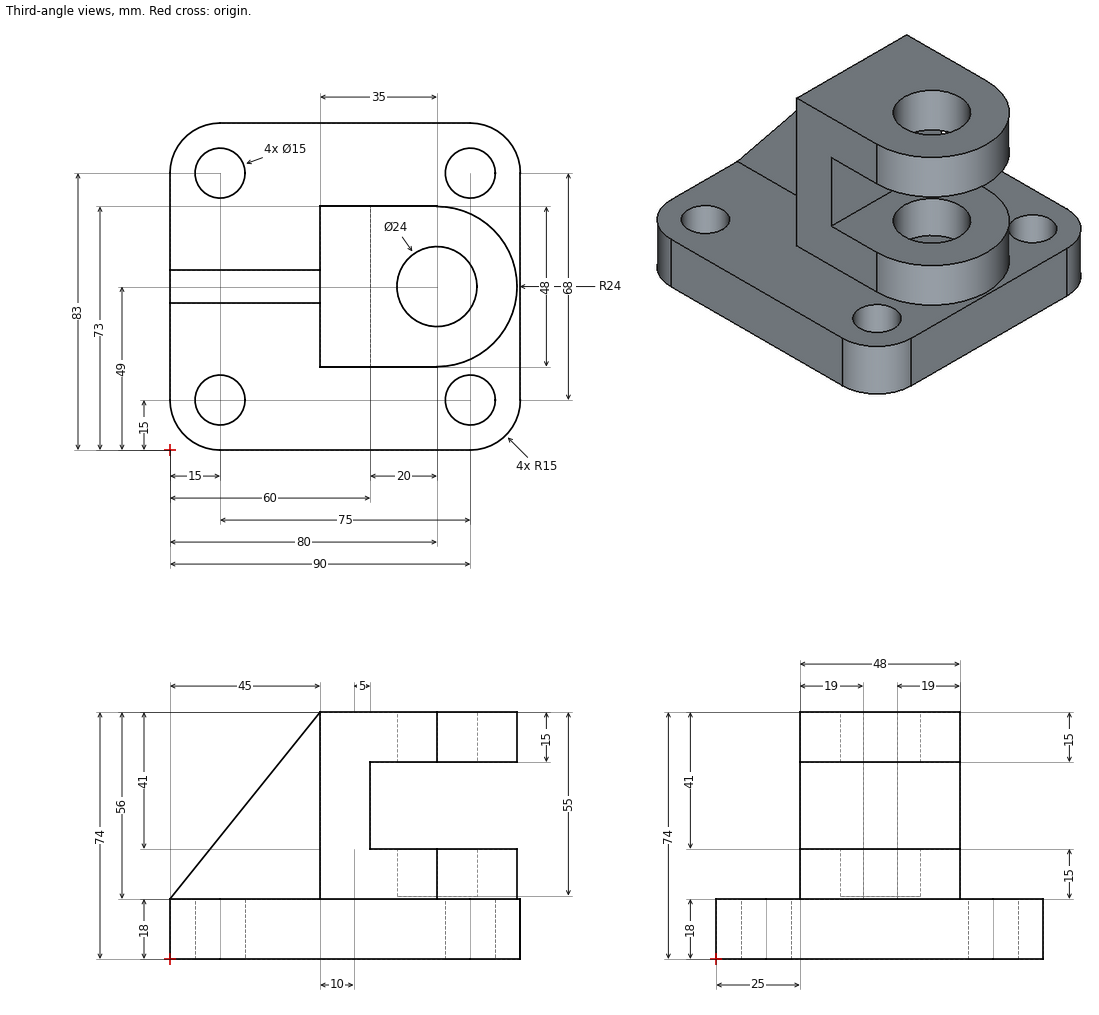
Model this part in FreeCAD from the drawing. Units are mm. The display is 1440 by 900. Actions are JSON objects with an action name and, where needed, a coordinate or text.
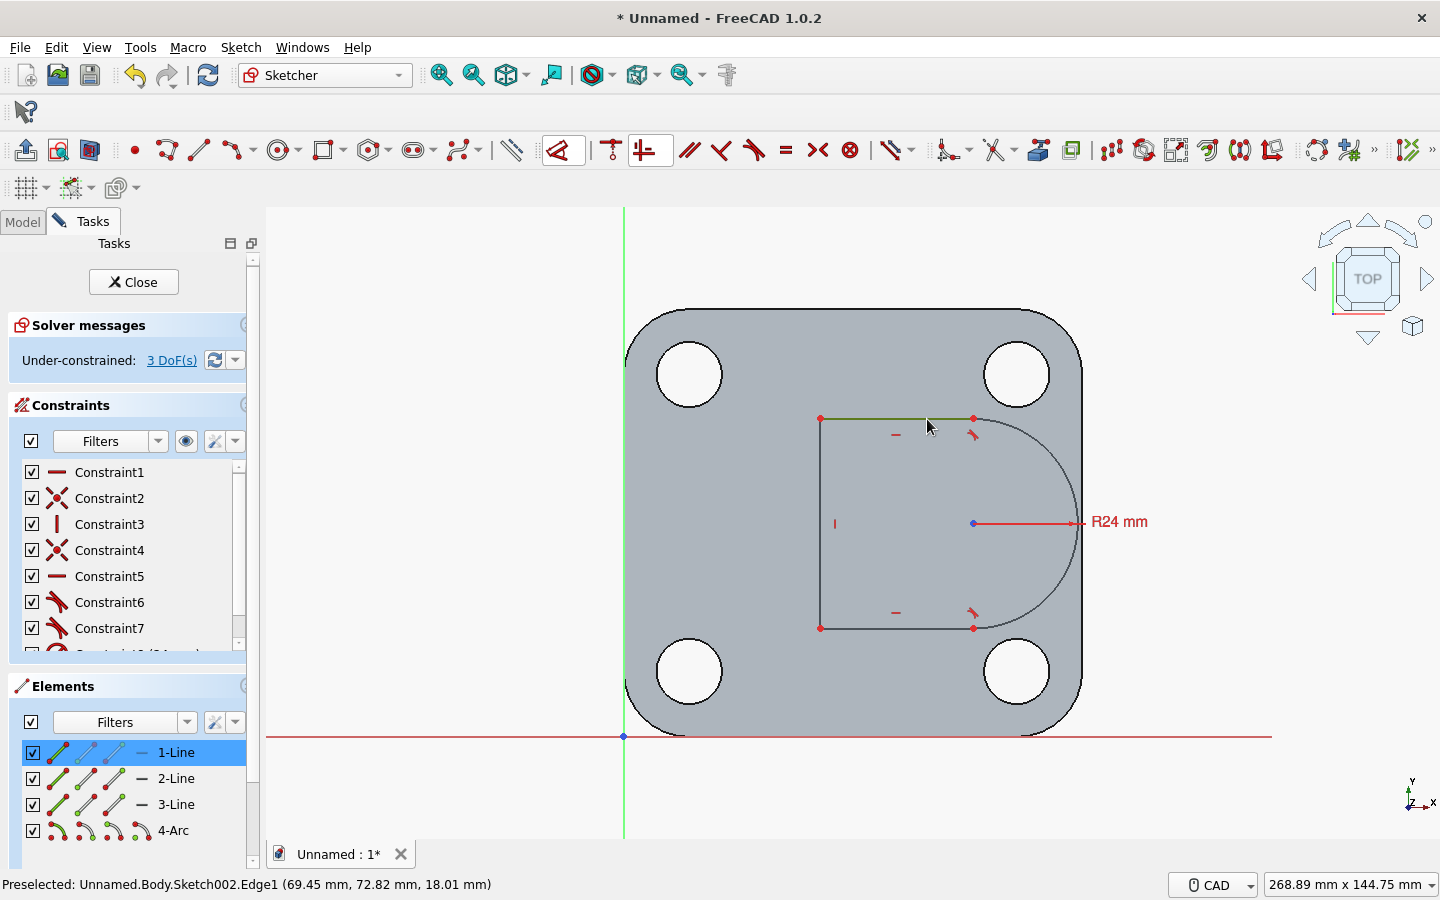
{"action": "key", "text": "l"}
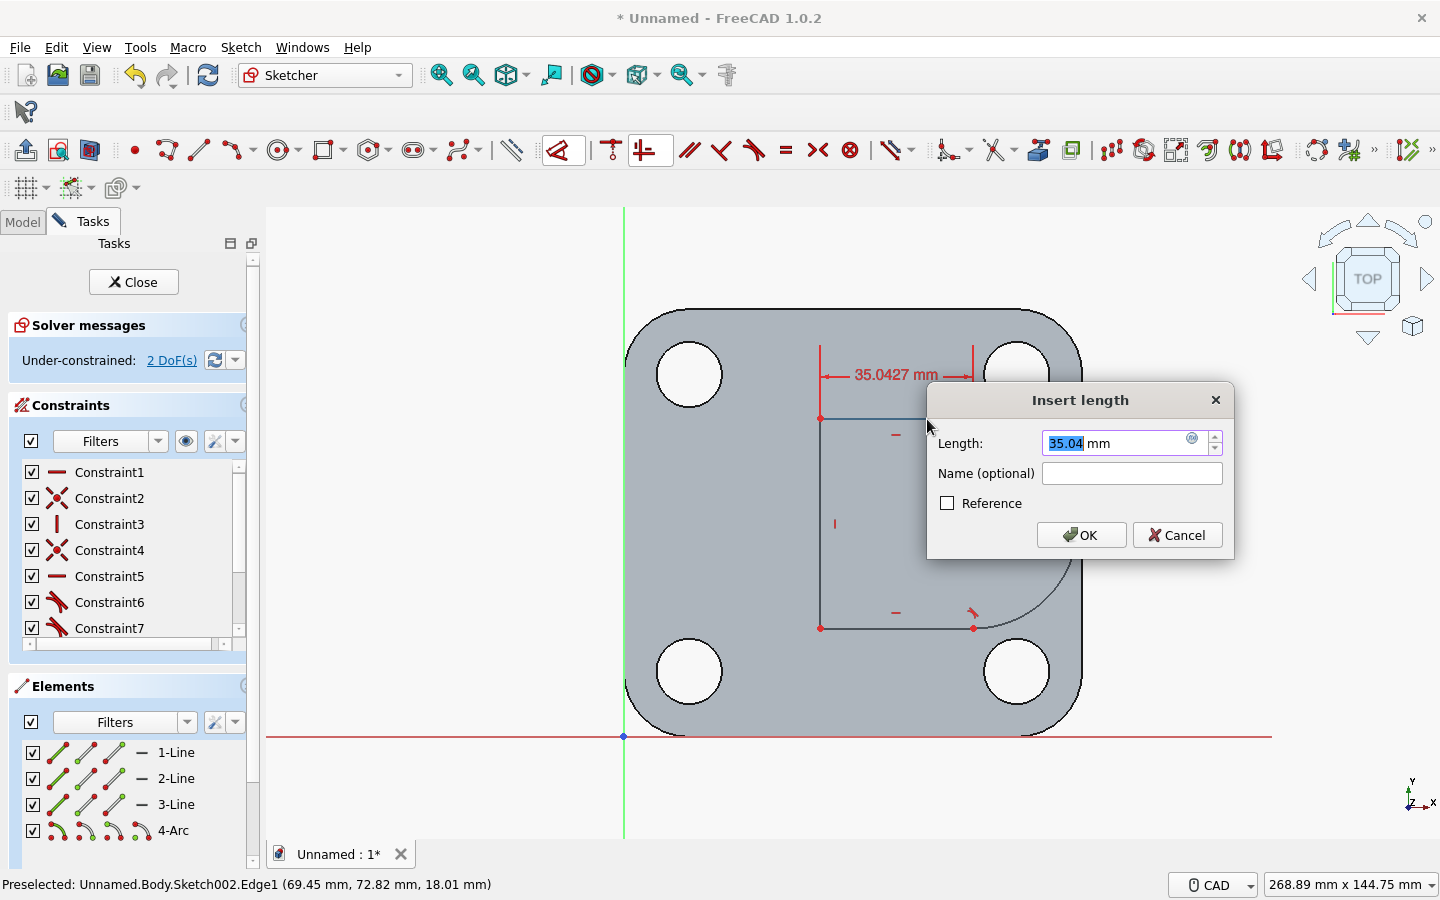
{"action": "type", "text": "35"}
{"action": "key", "text": "Return"}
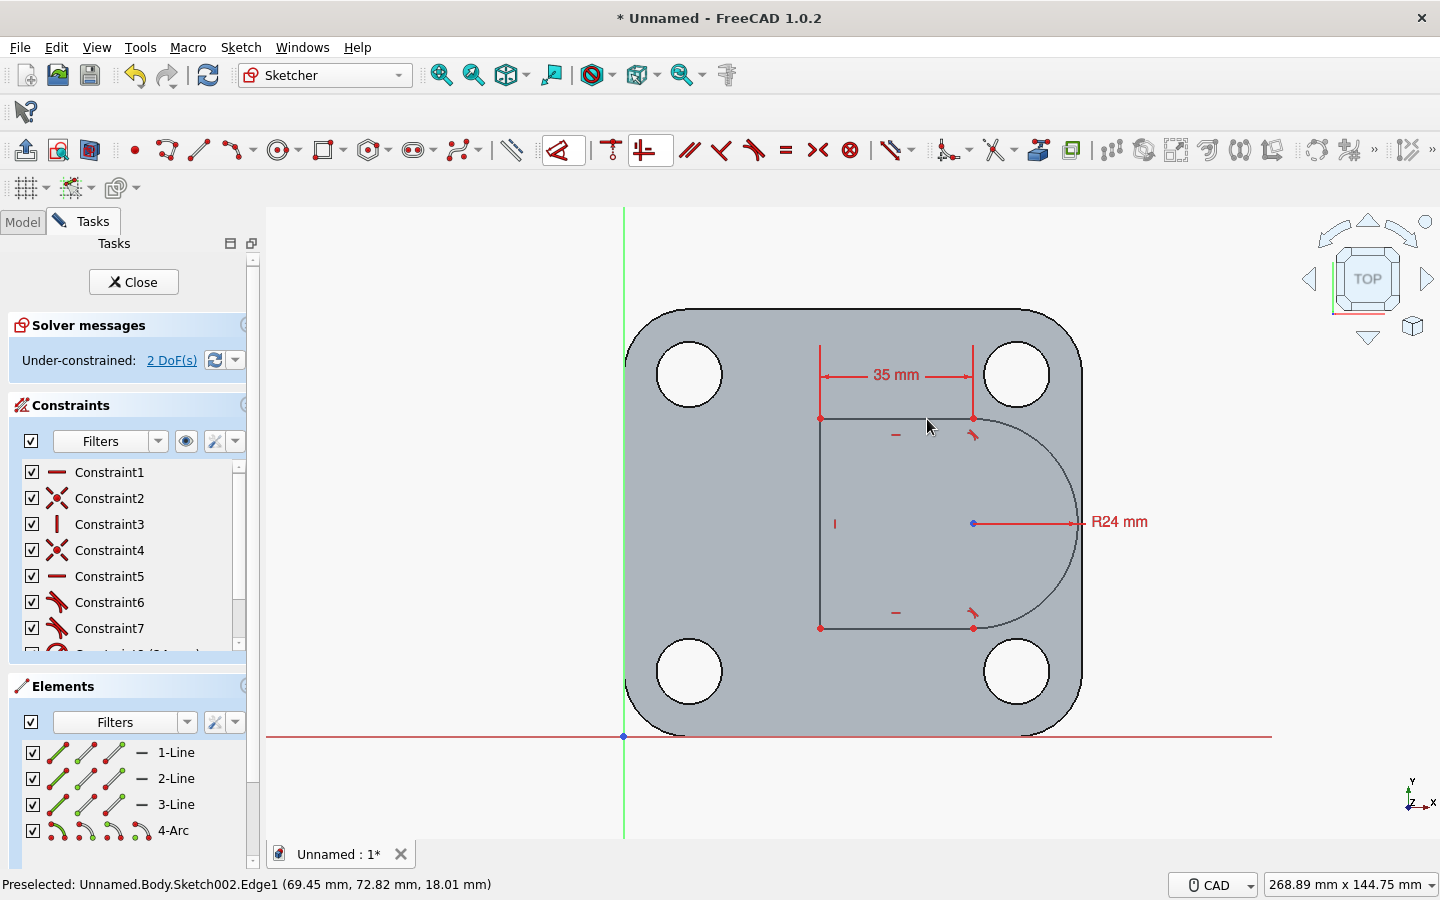
{"action": "left_click", "coordinate": [973, 419]}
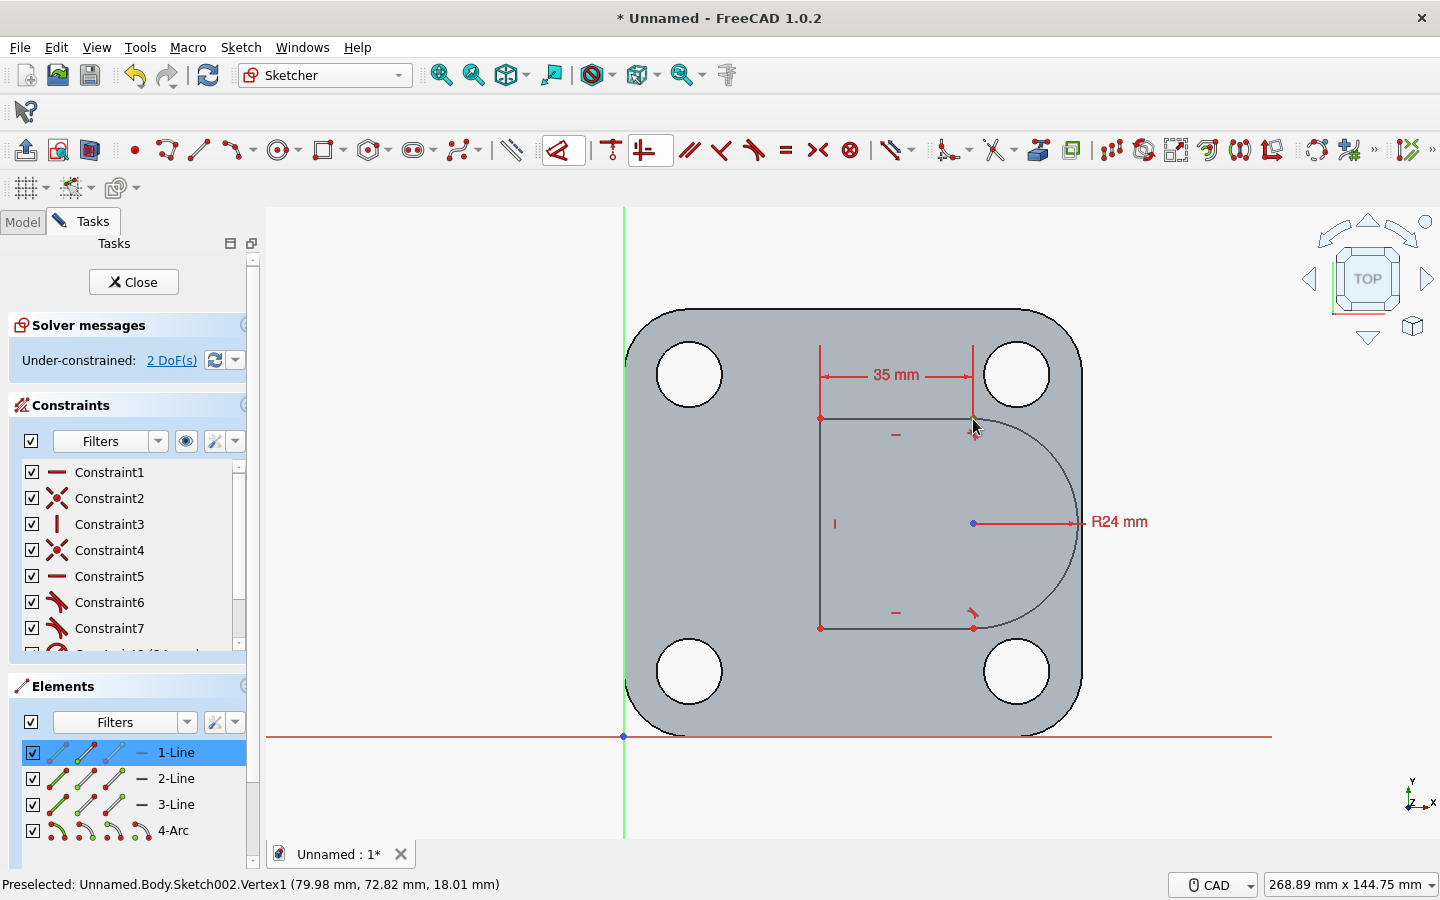
{"action": "left_click", "coordinate": [580, 150]}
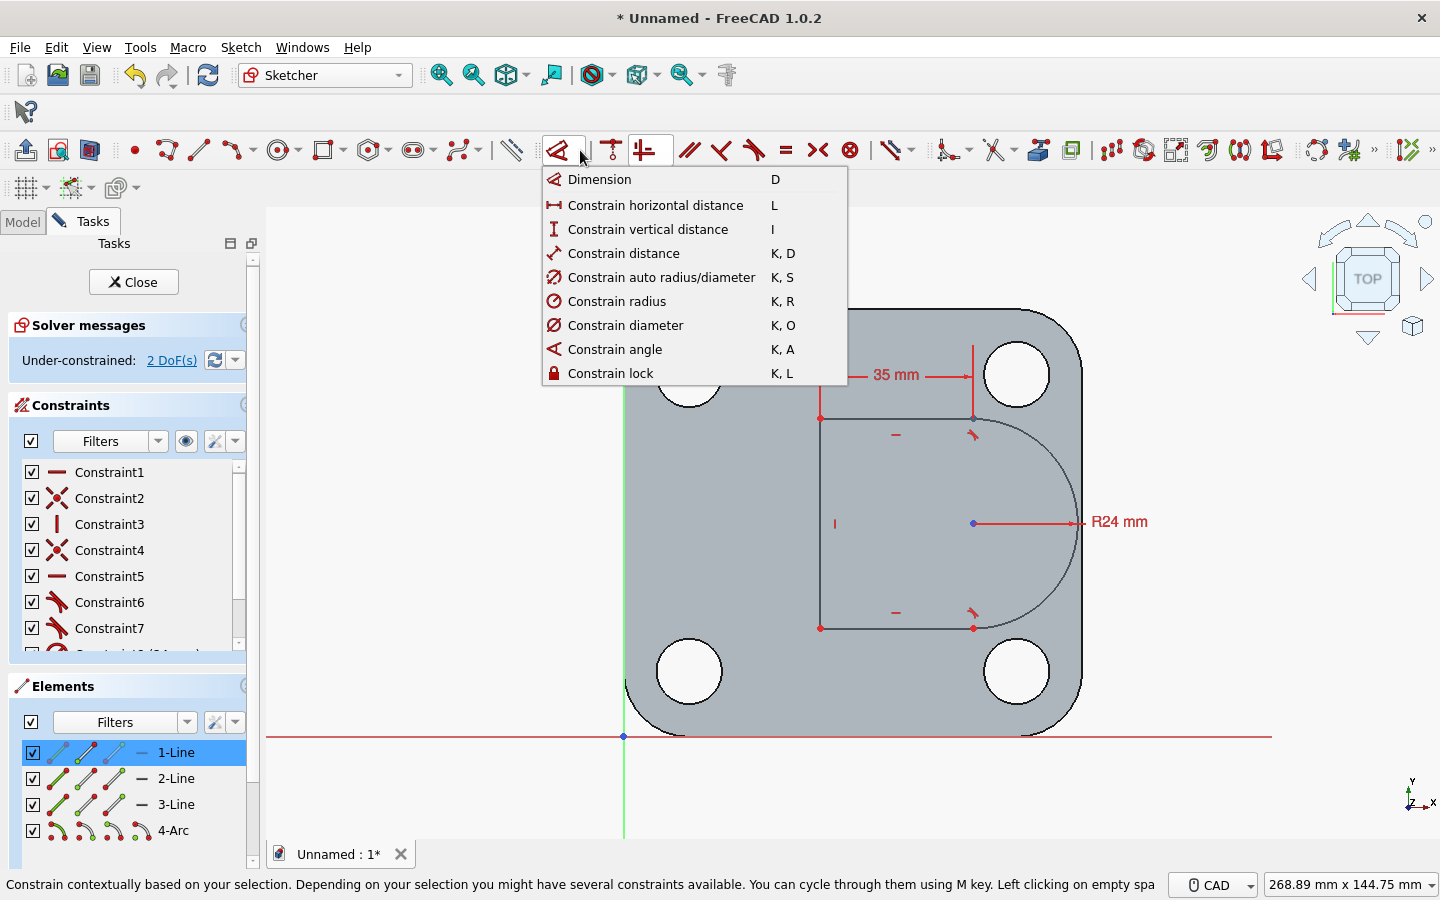
{"action": "left_click", "coordinate": [695, 205]}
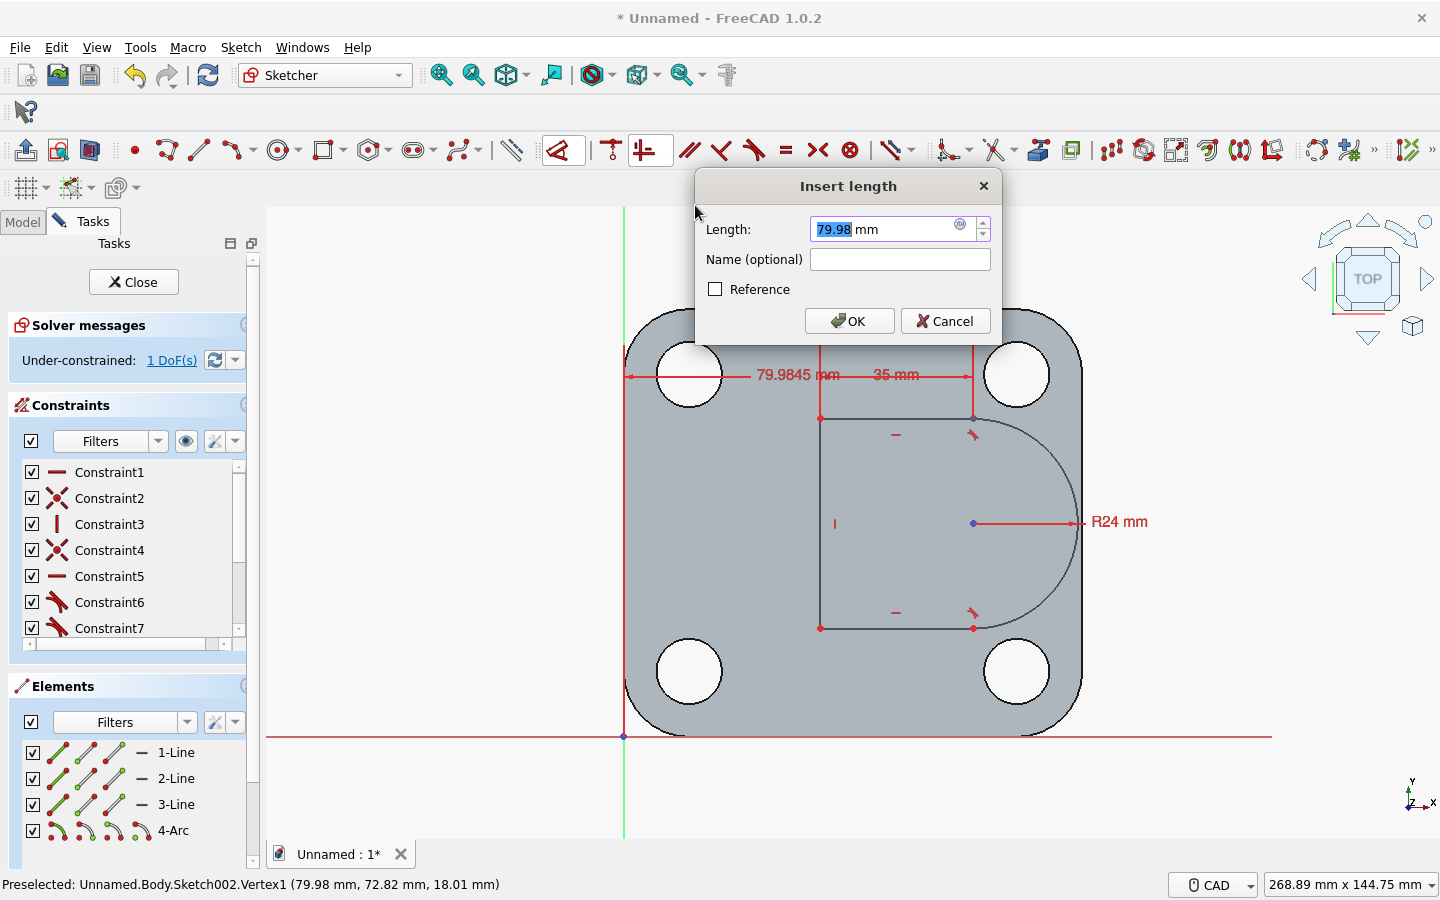
{"action": "type", "text": "80"}
{"action": "key", "text": "Return"}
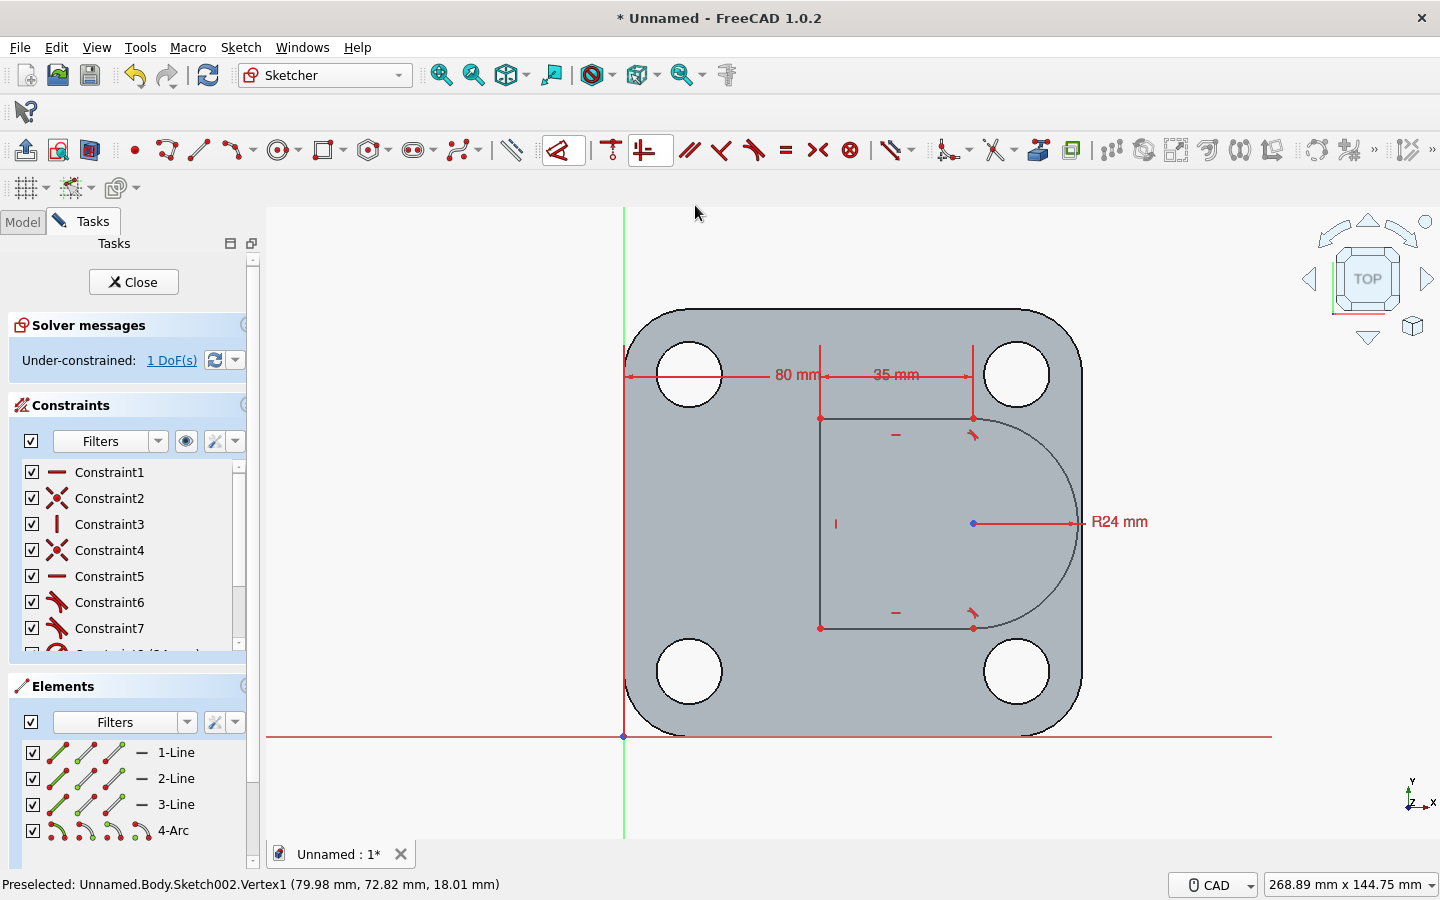
{"action": "left_click", "coordinate": [973, 419]}